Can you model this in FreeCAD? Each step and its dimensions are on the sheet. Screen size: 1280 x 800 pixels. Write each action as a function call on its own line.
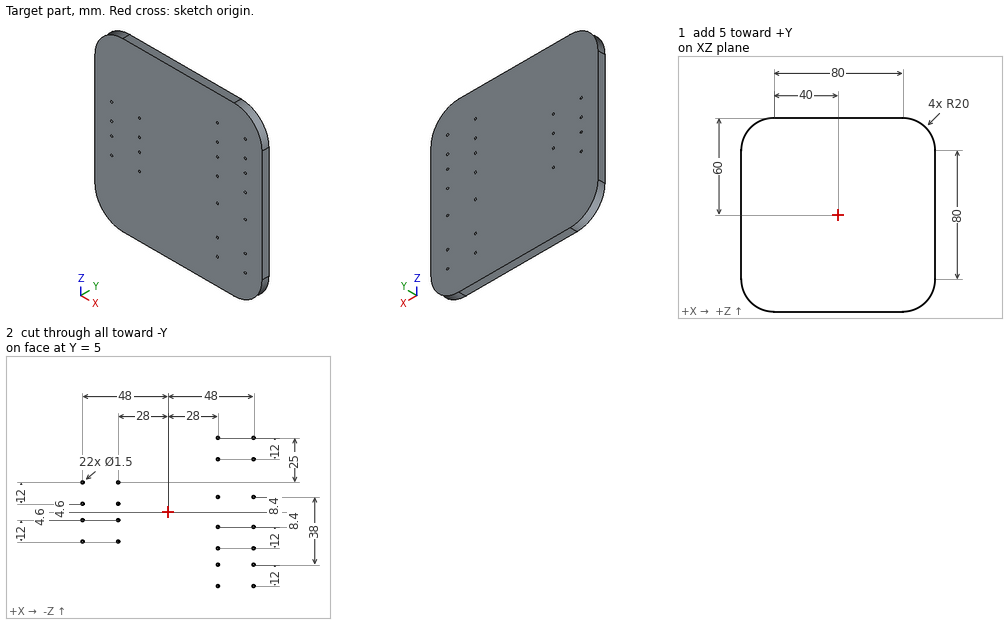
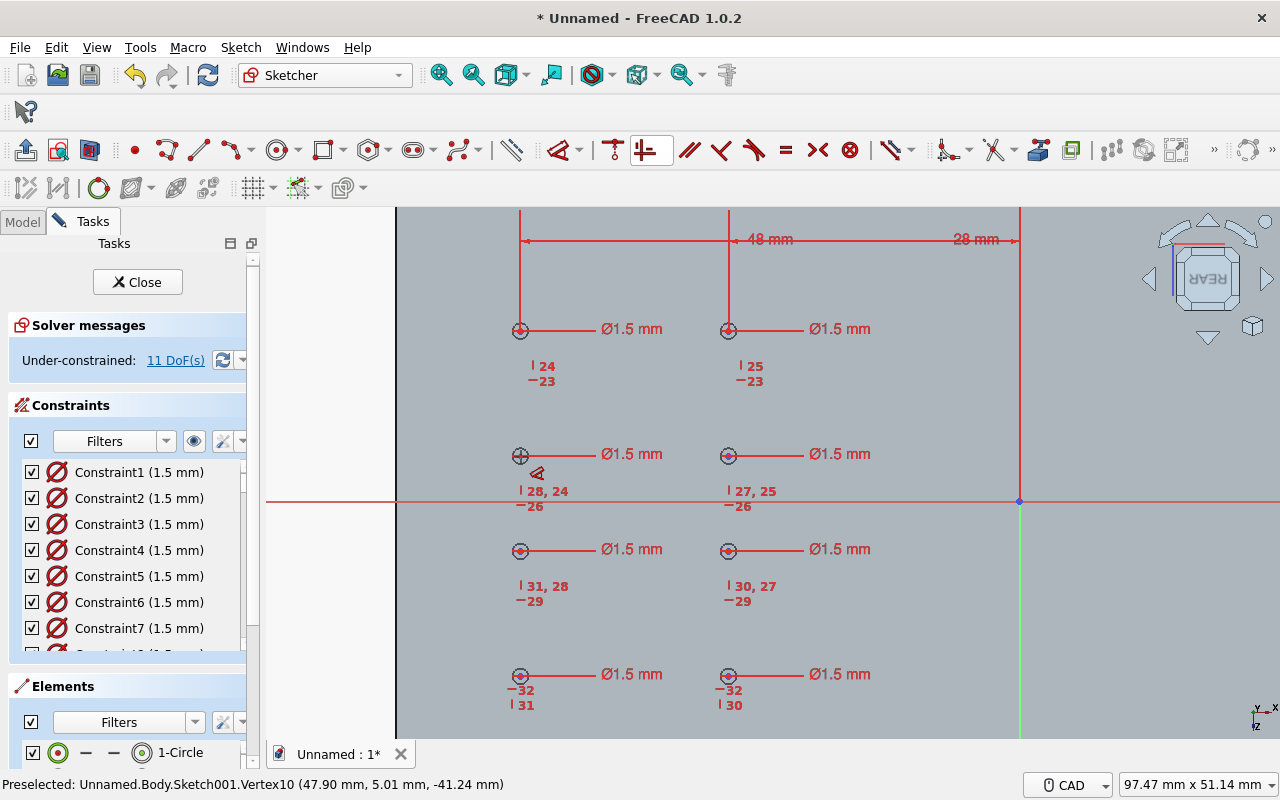
click(520, 456)
click(486, 479)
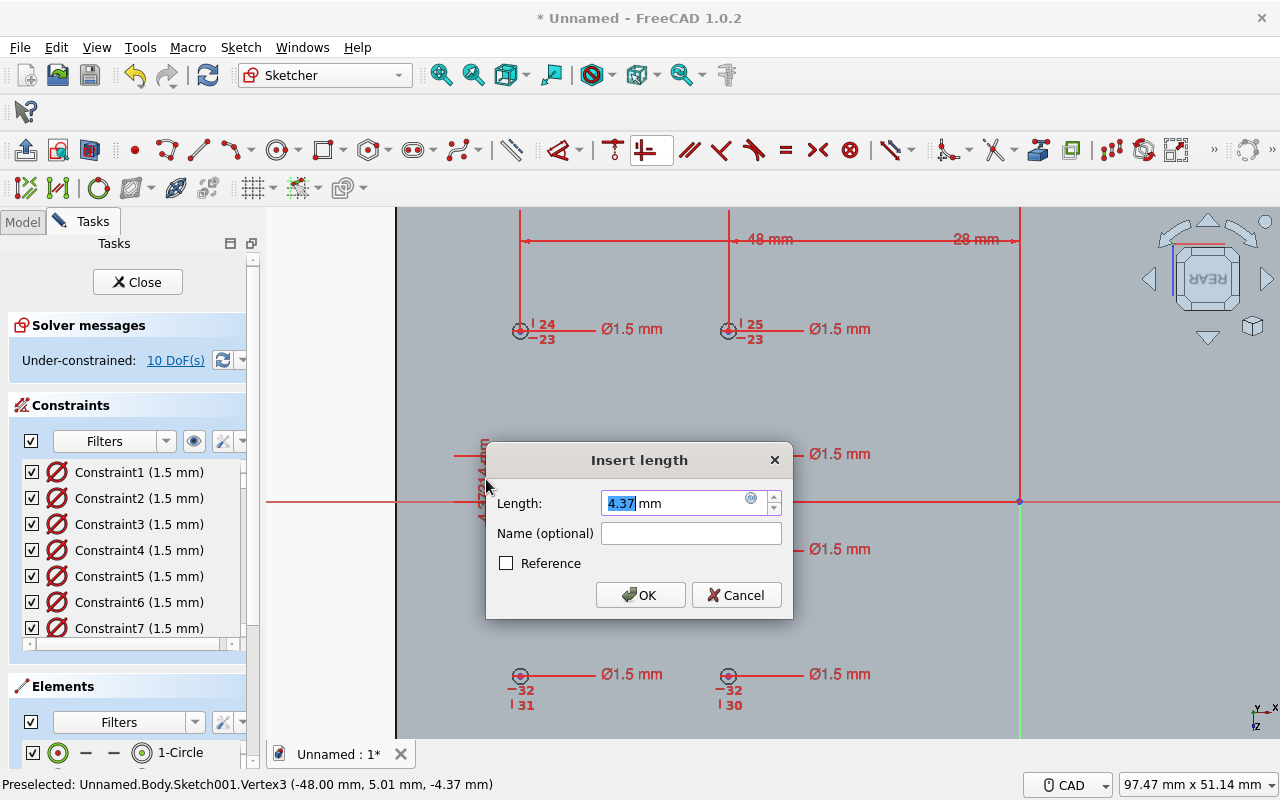
text(4.6)
key(Return)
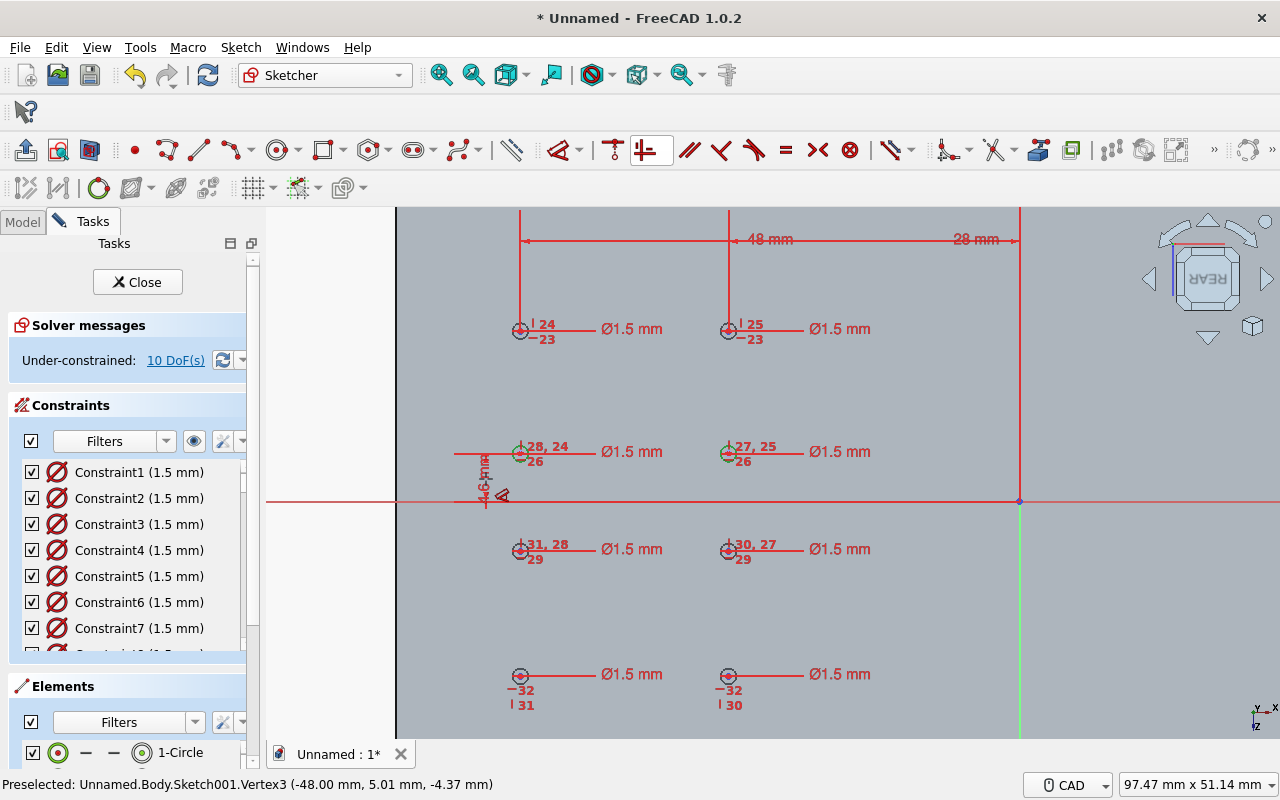
click(729, 551)
click(695, 527)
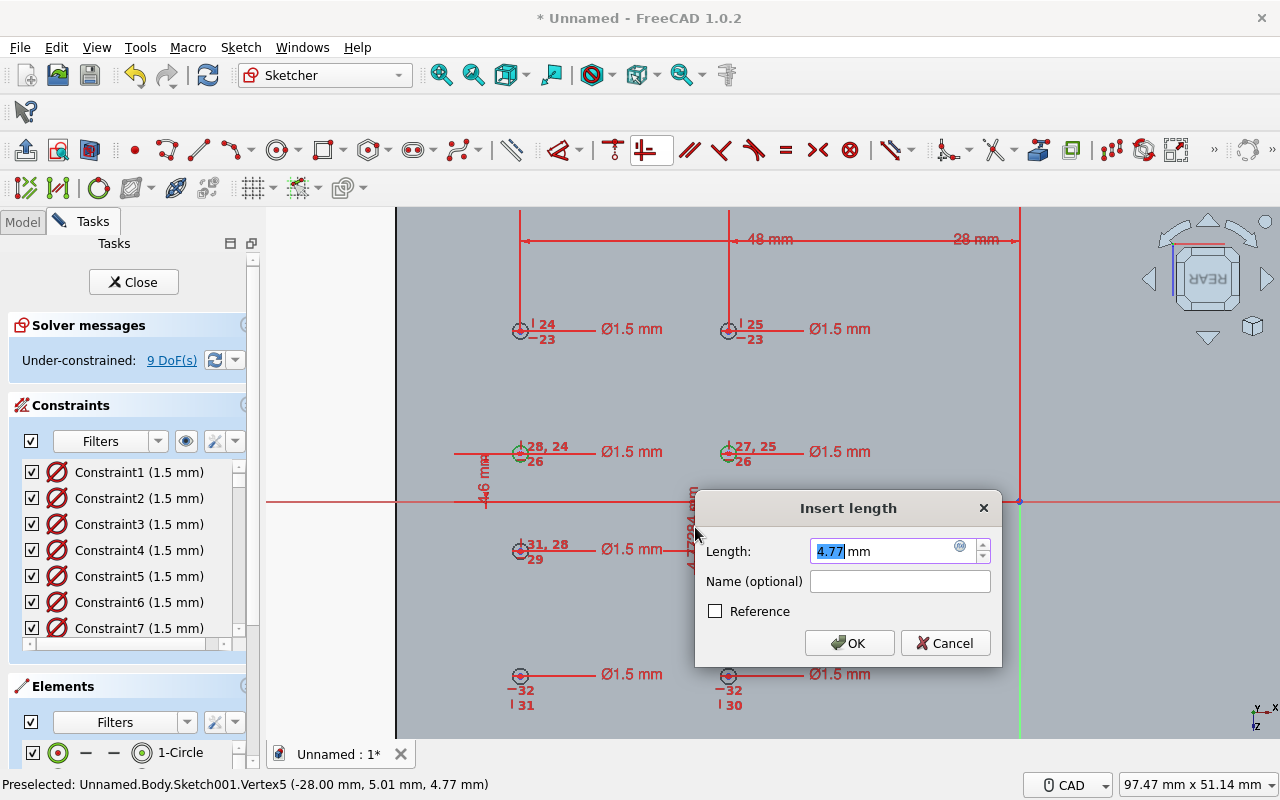
text(4.6)
key(Return)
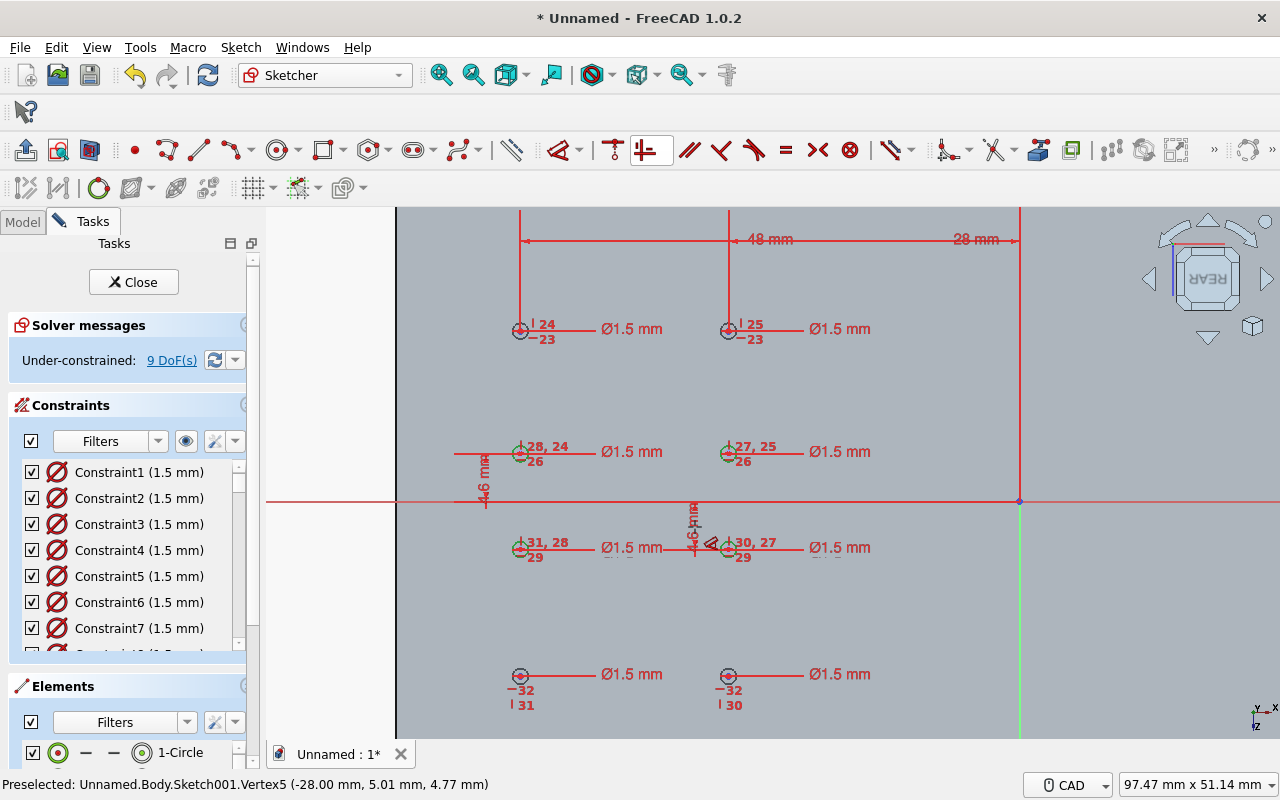
scroll(521, 456, down, 5)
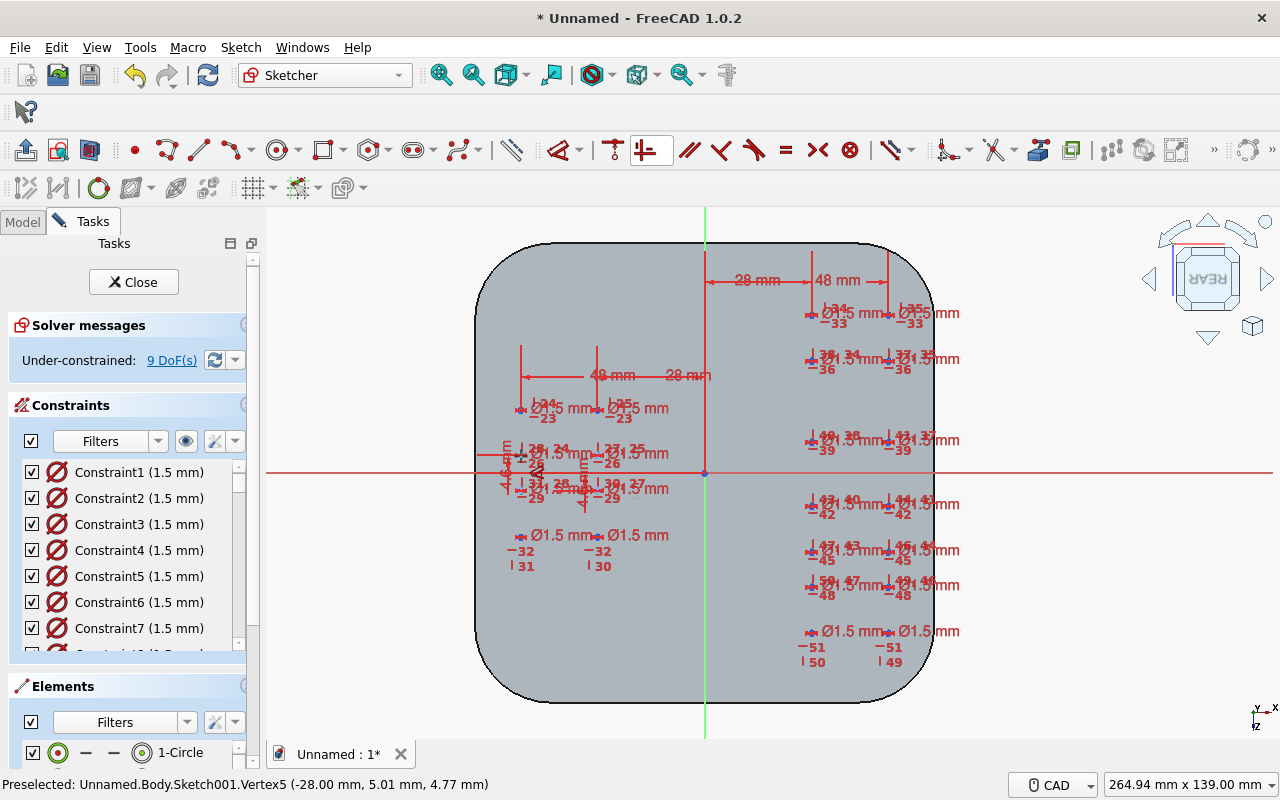
scroll(888, 442, up, 2)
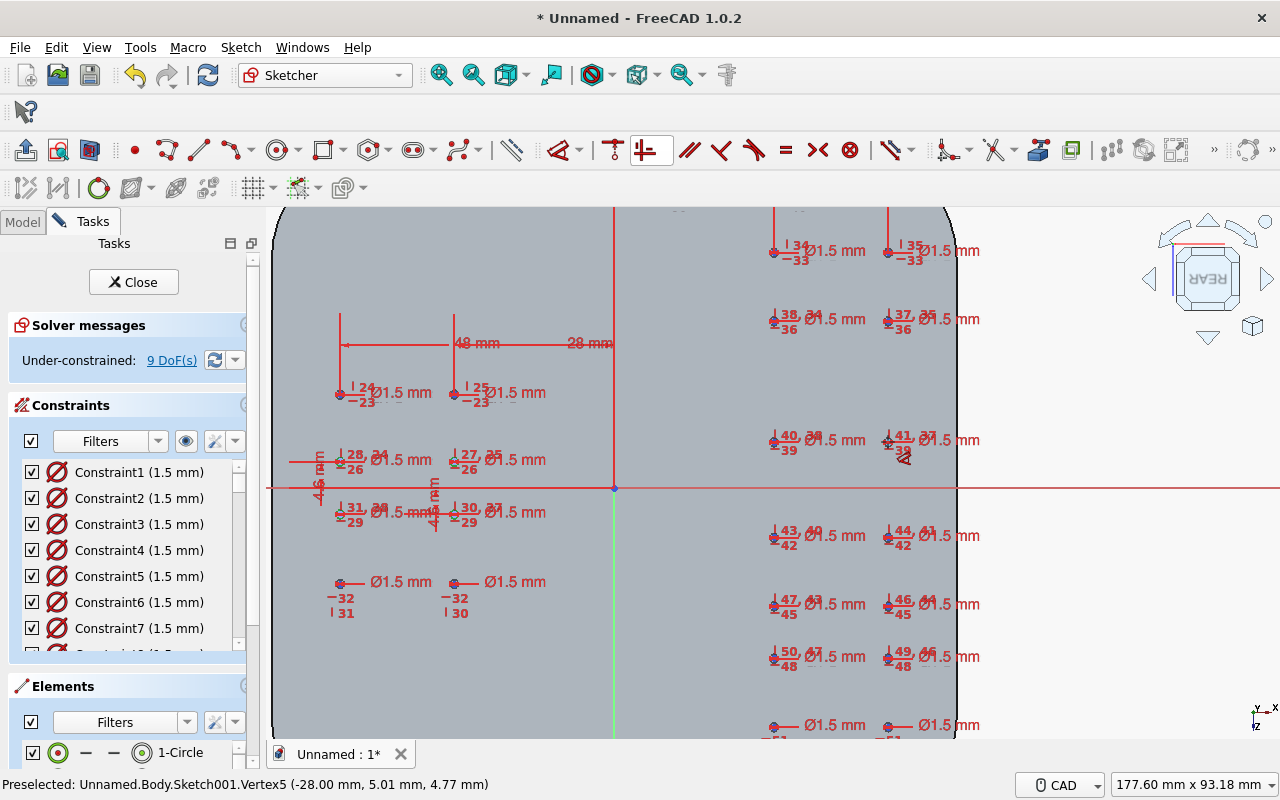
click(888, 442)
click(922, 465)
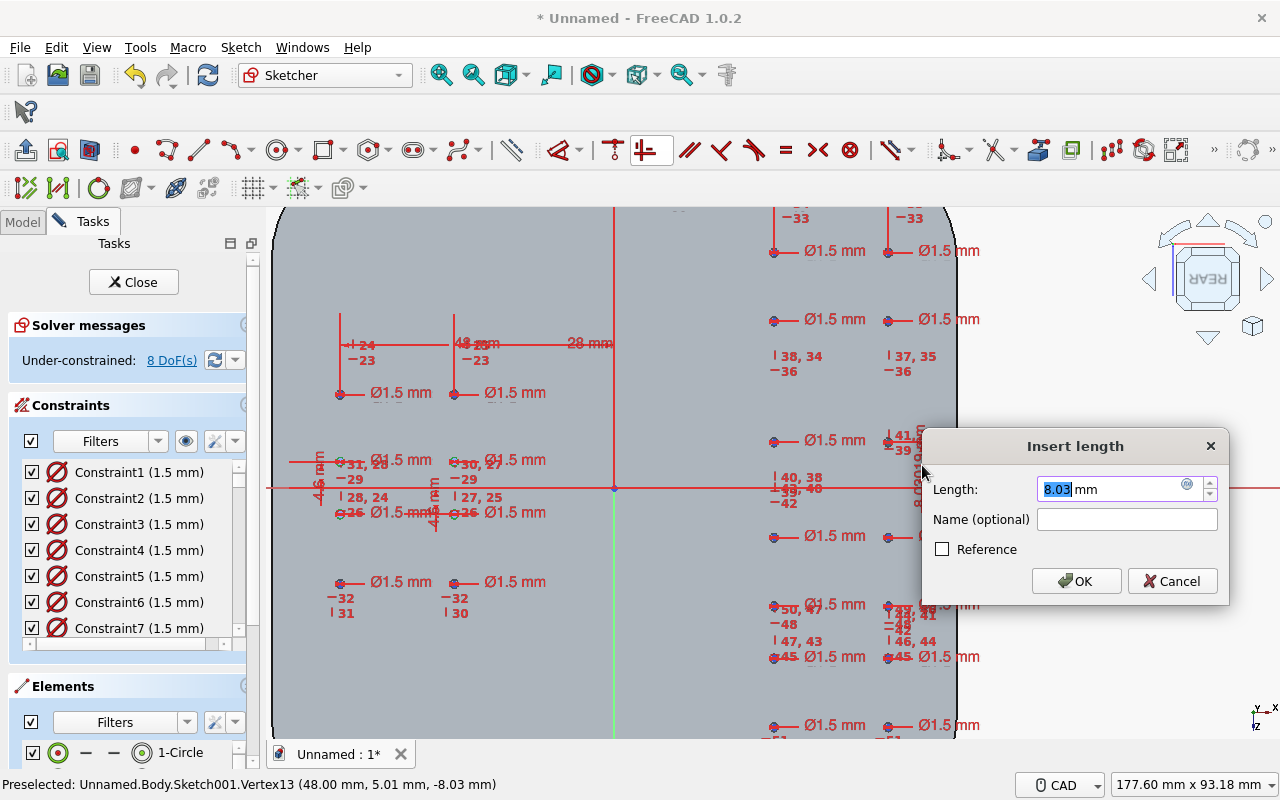
text(8.4)
key(Return)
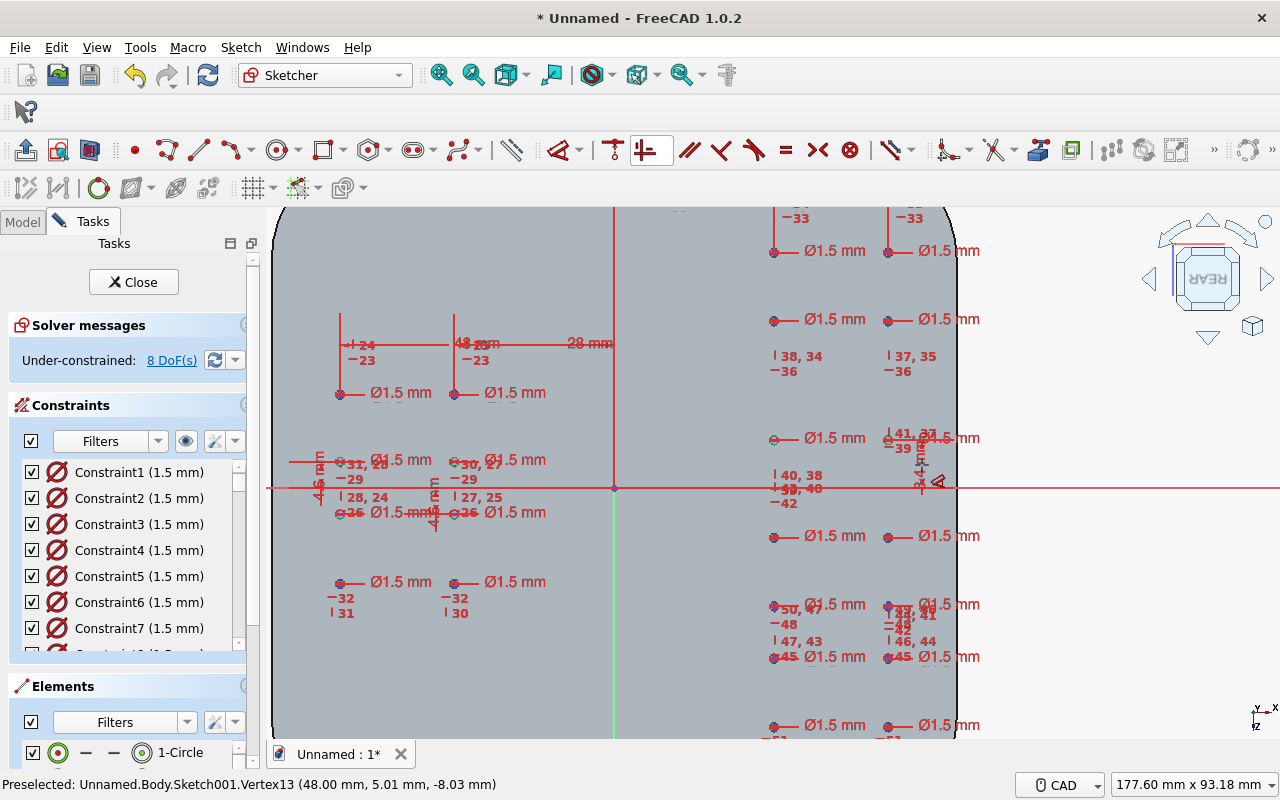
click(774, 538)
click(808, 513)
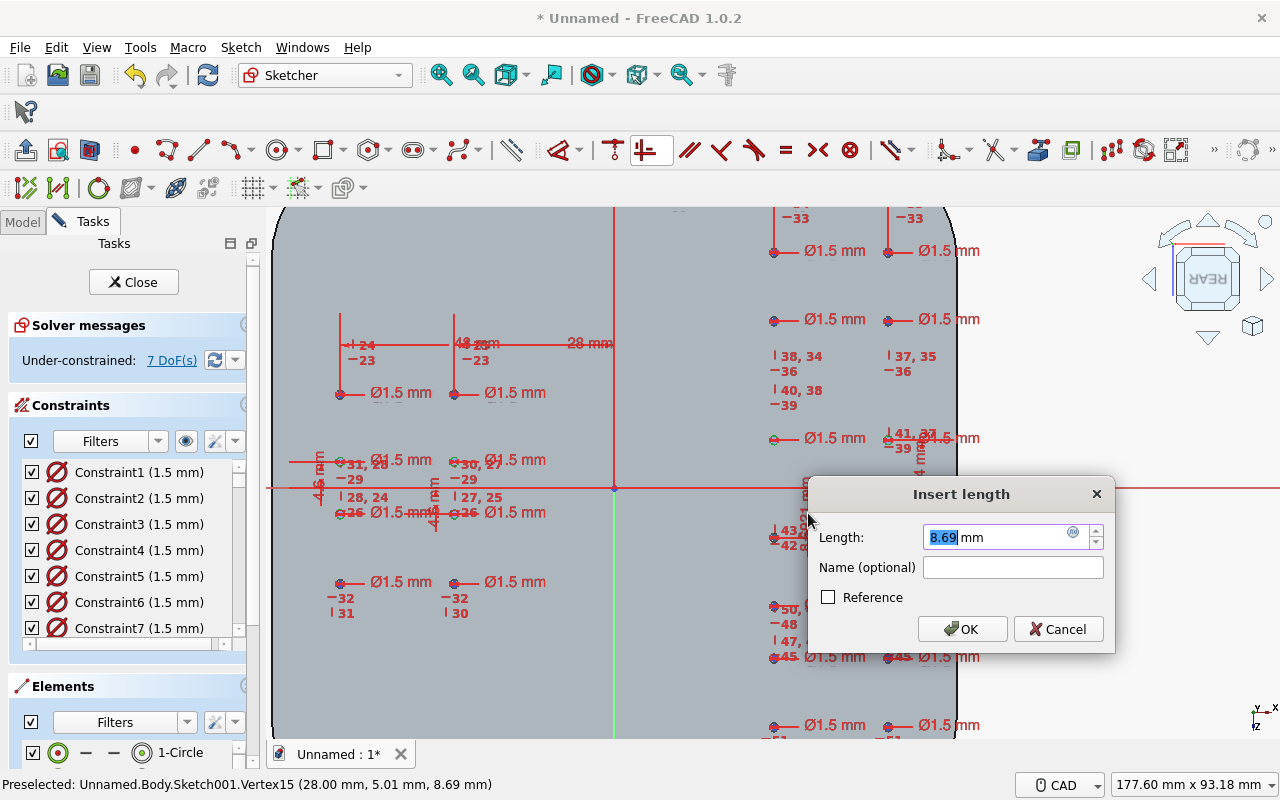
text(8.4)
key(Return)